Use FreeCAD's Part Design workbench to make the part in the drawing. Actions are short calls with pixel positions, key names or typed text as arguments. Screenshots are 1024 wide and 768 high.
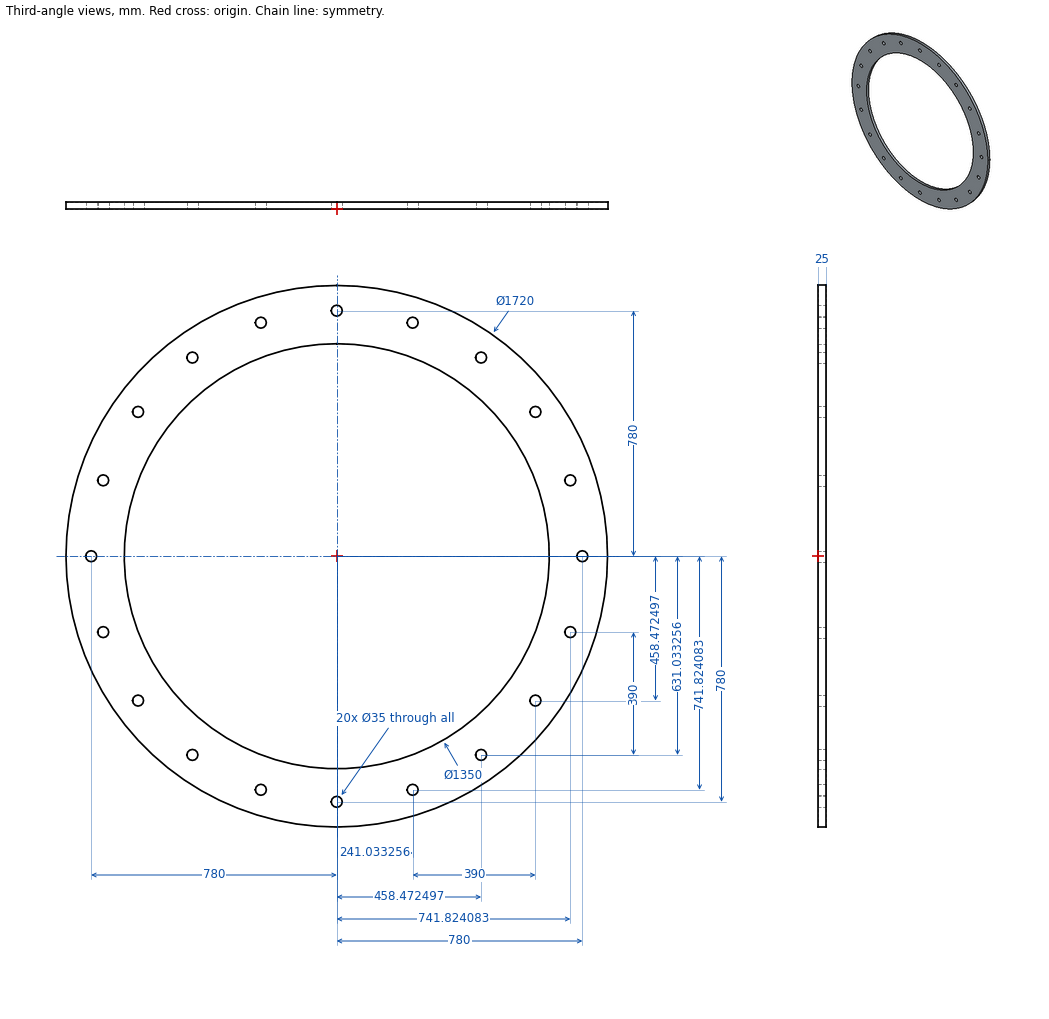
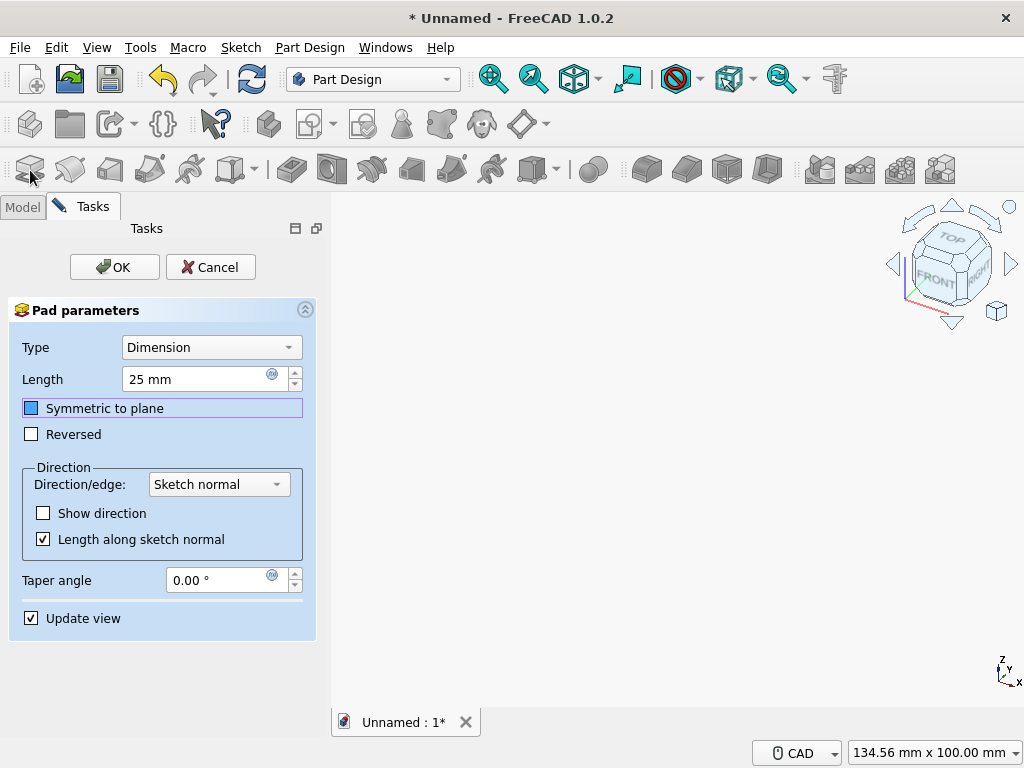
click(30, 434)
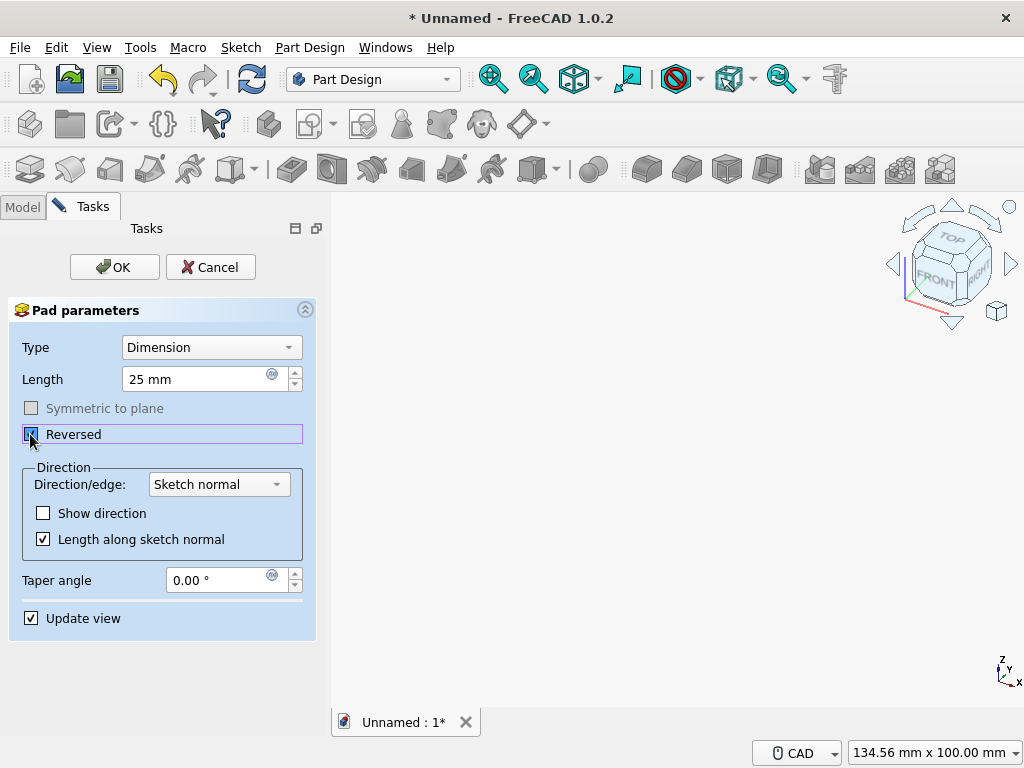
click(115, 267)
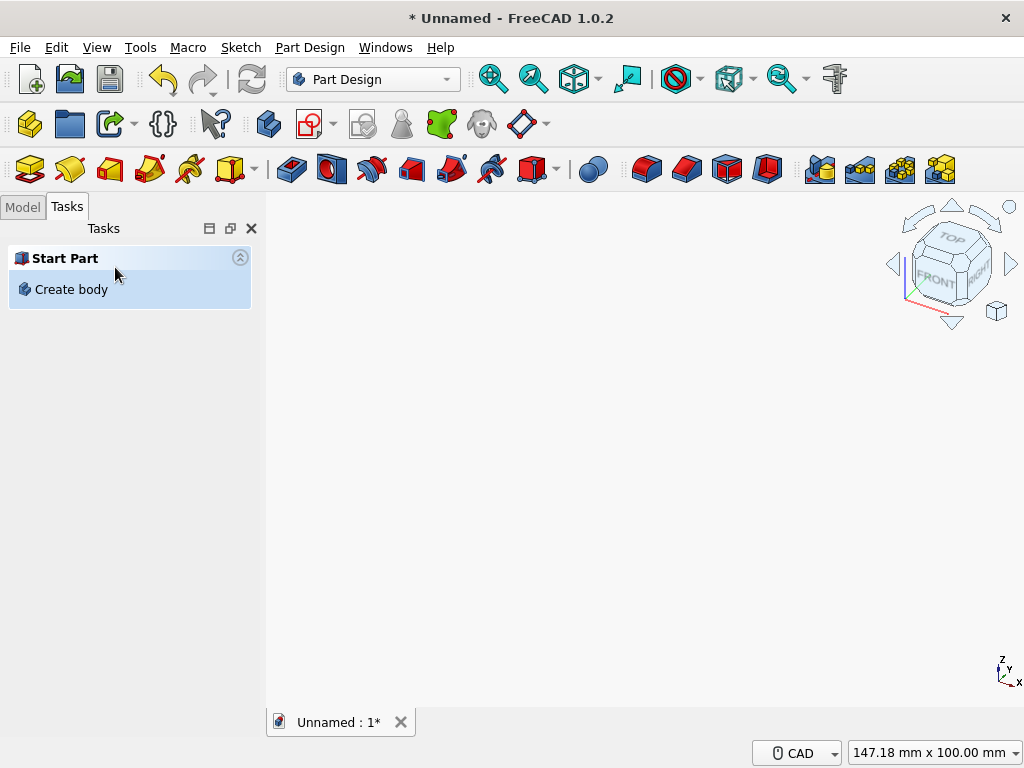
key(v)
key(f)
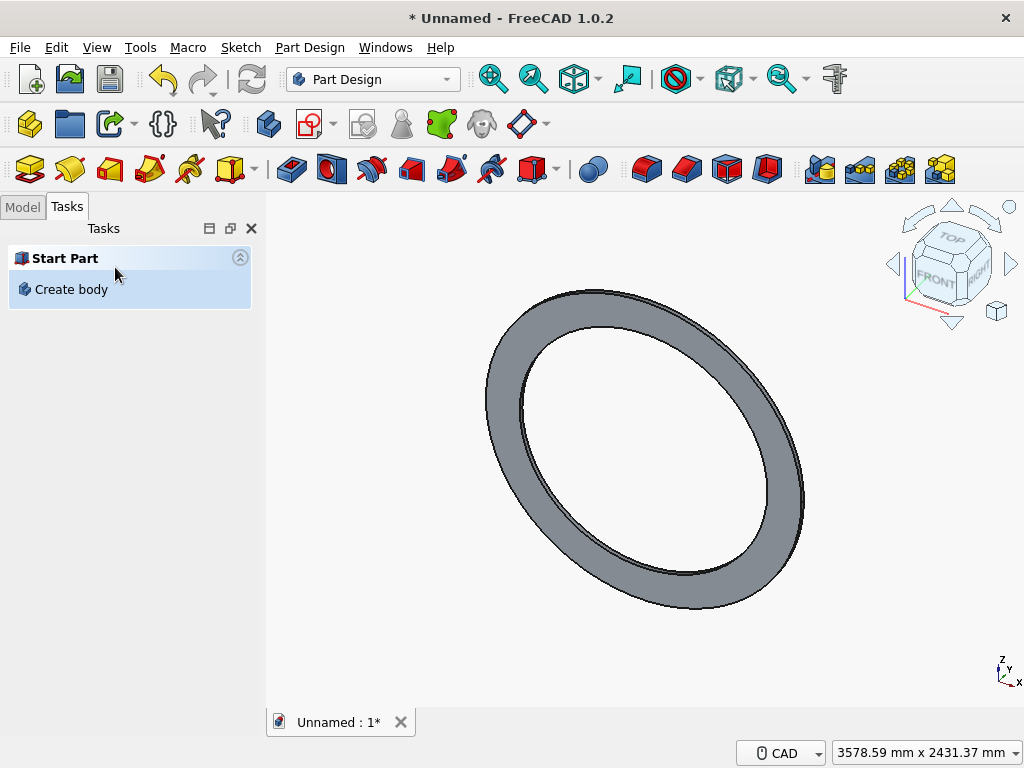
key(4)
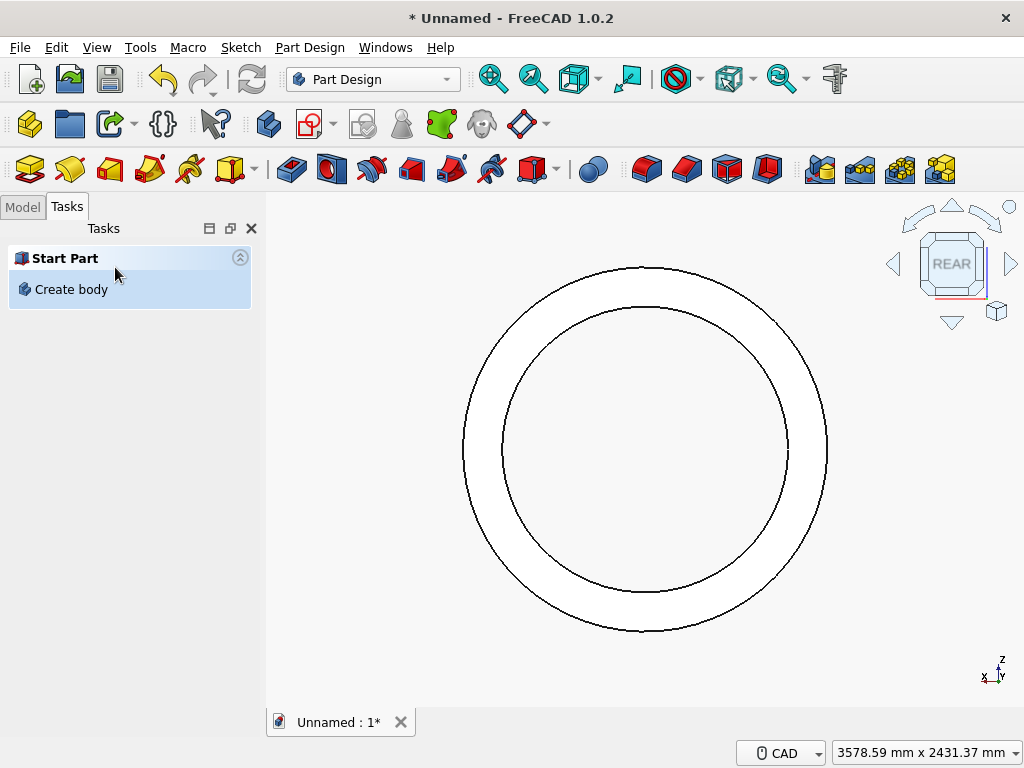
click(801, 501)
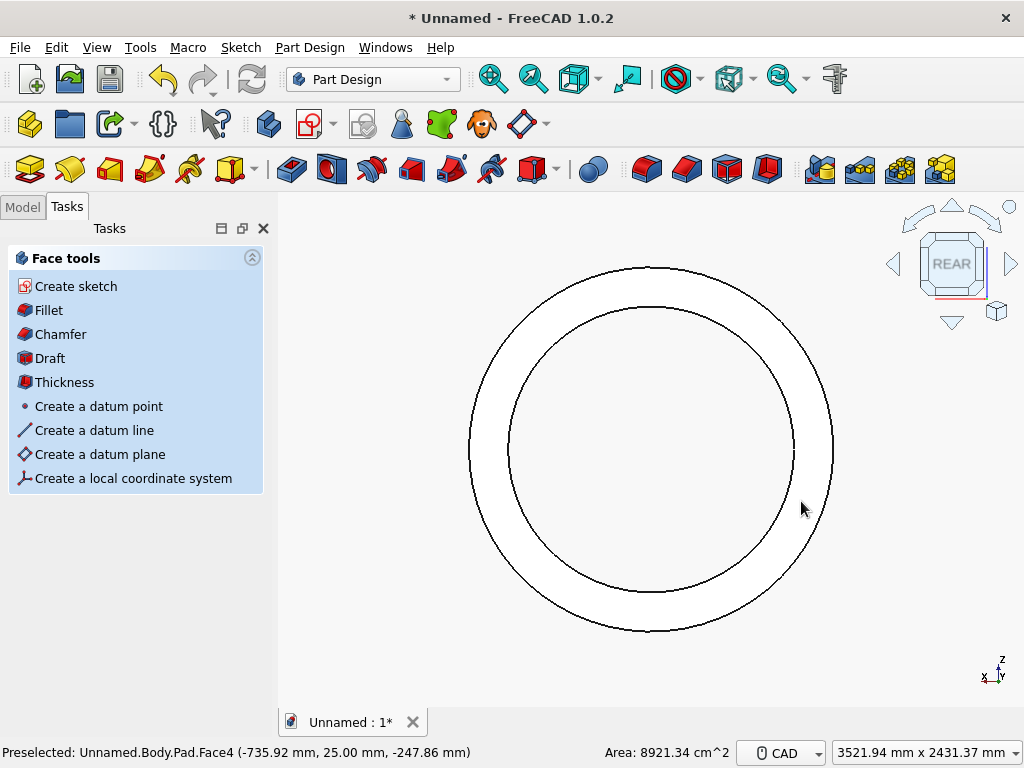
click(310, 124)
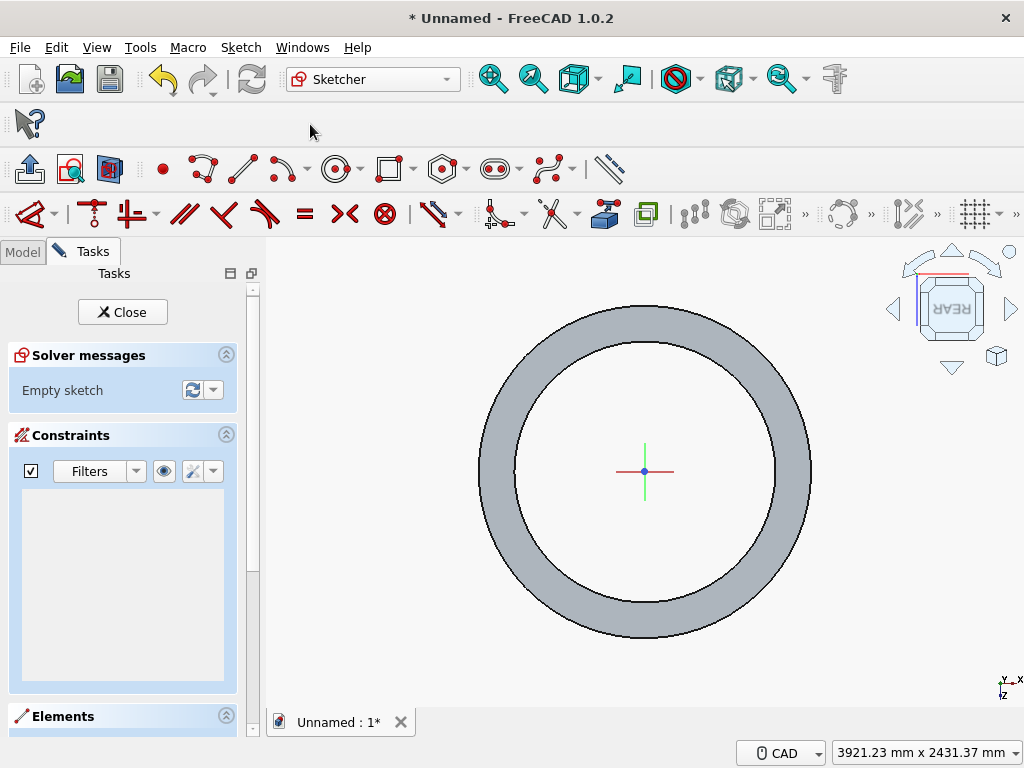
key(g)
key(c)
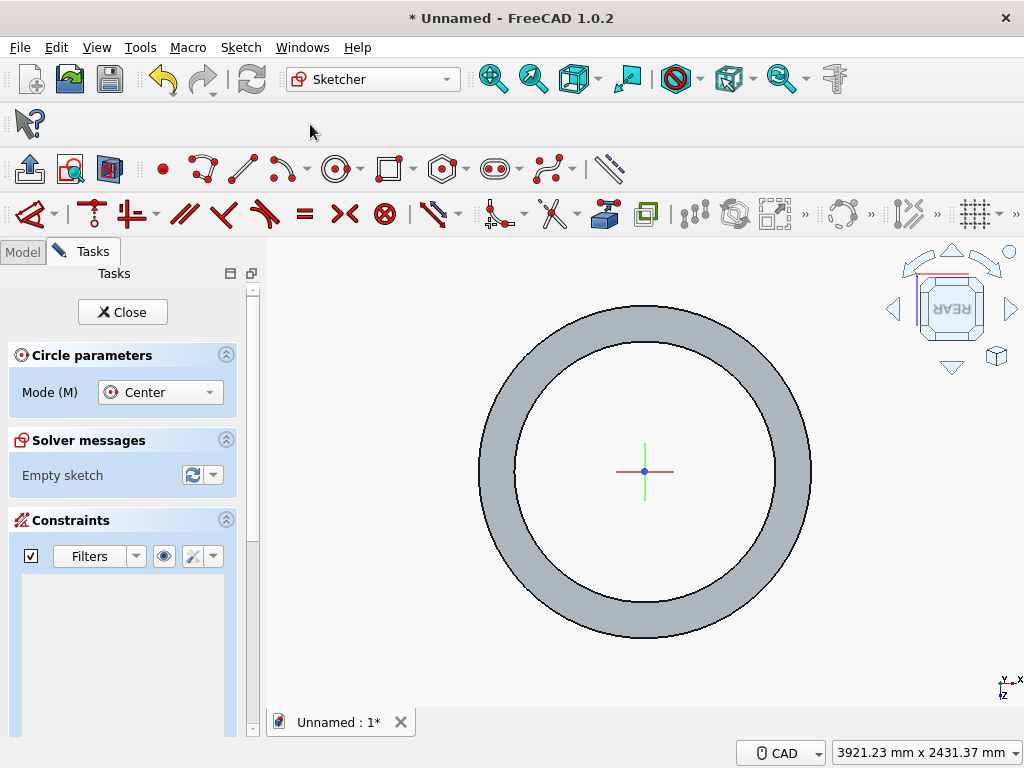
scroll(645, 321, up, 10)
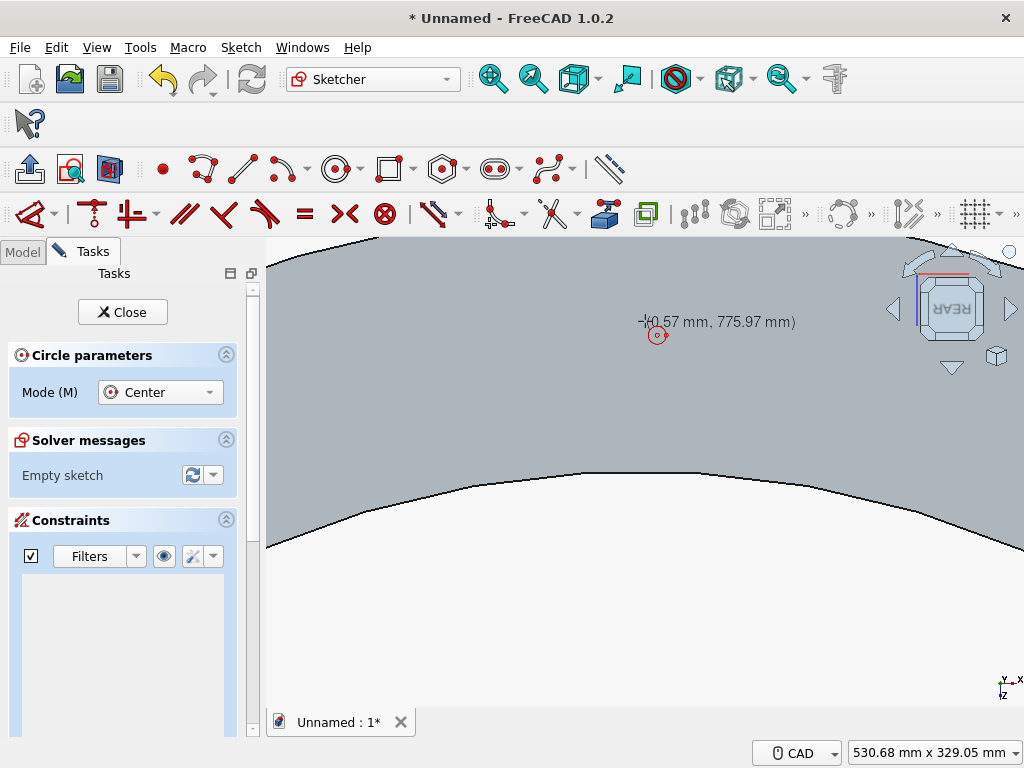
scroll(566, 321, down, 10)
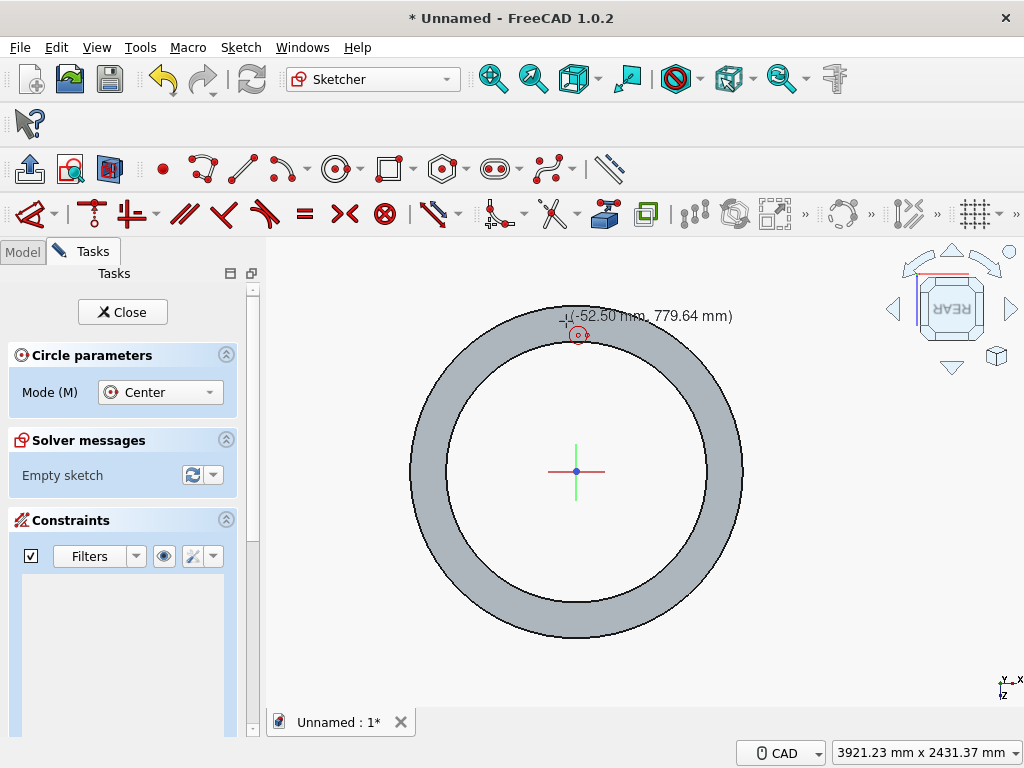
click(576, 321)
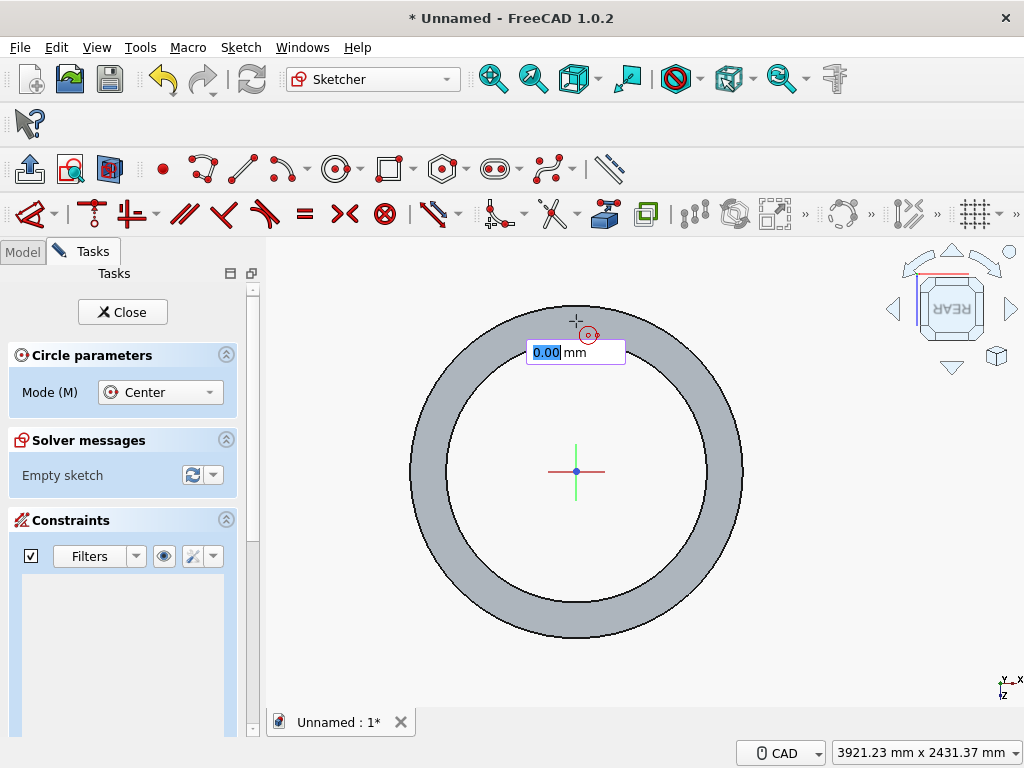
scroll(580, 320, up, 9)
move(576, 319)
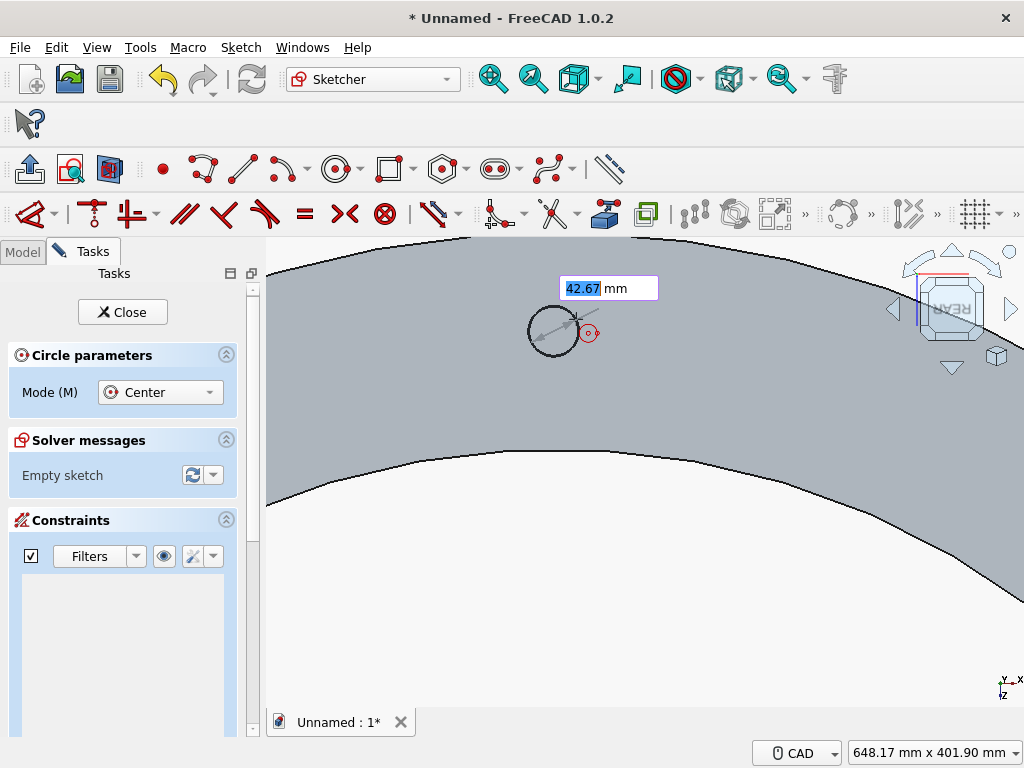
text(35)
key(Return)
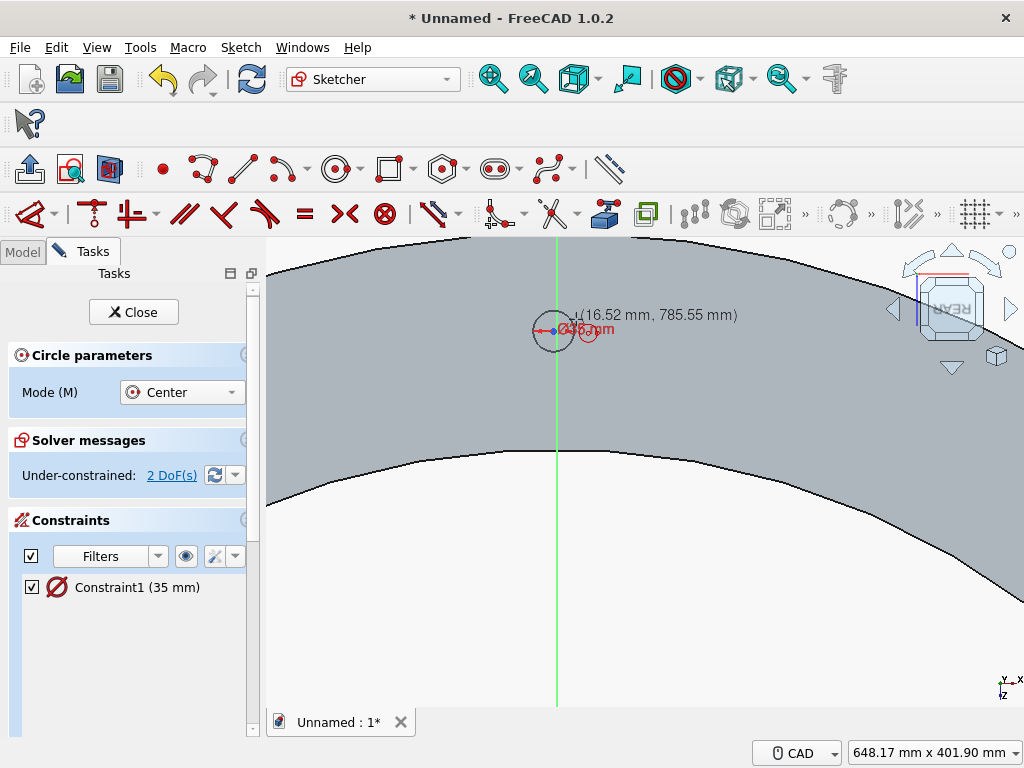
scroll(580, 320, down, 9)